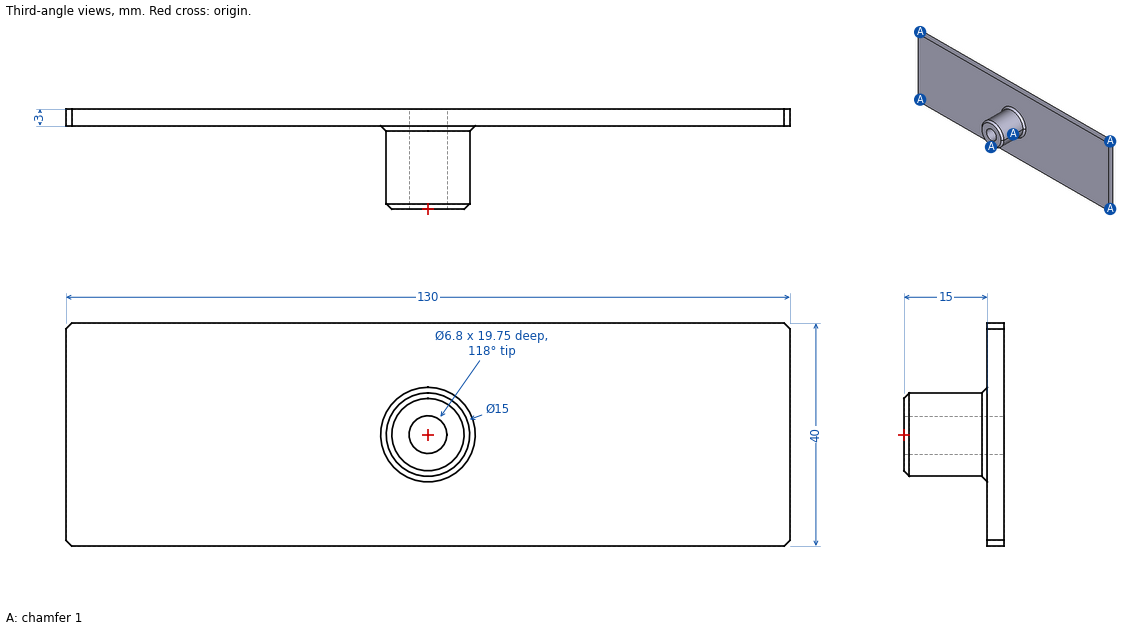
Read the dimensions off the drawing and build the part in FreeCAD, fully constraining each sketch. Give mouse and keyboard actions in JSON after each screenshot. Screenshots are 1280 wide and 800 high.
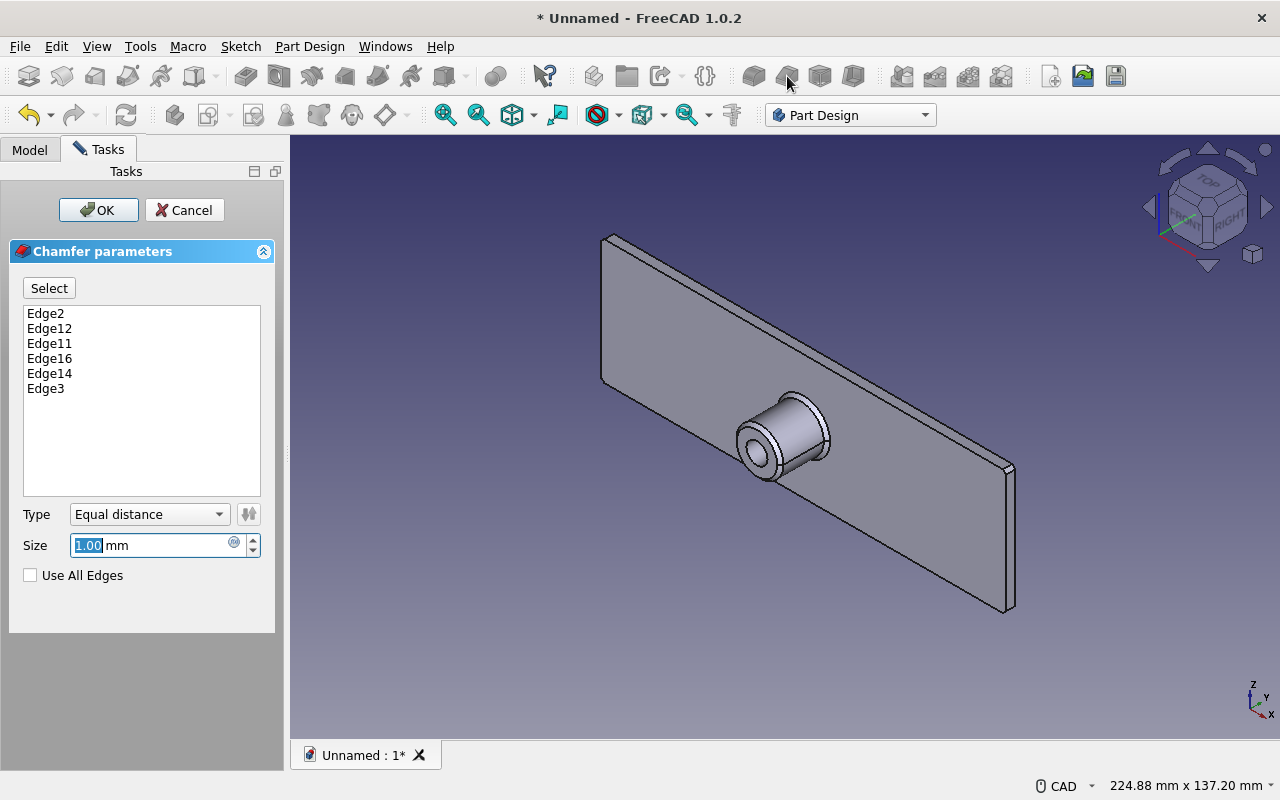
{"action": "type", "text": "1"}
{"action": "key", "text": "Tab"}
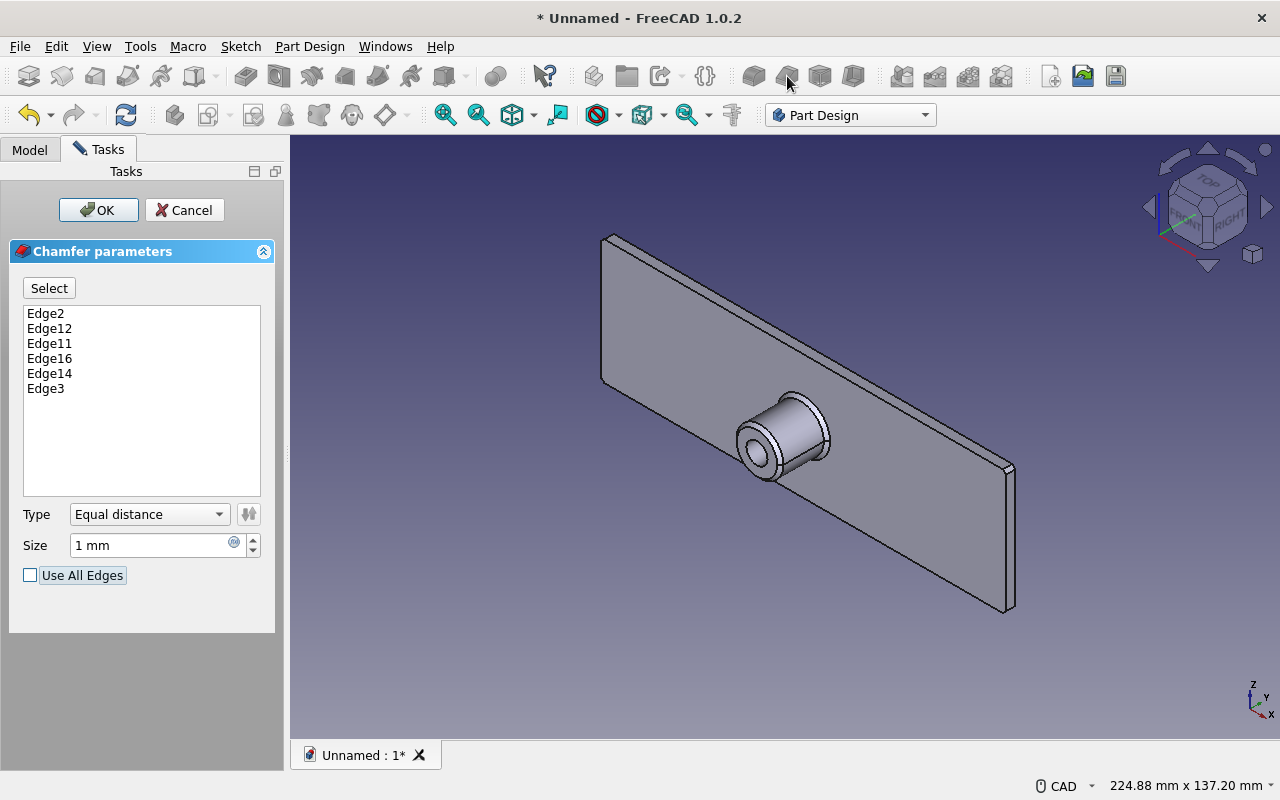
{"action": "left_click", "coordinate": [99, 210]}